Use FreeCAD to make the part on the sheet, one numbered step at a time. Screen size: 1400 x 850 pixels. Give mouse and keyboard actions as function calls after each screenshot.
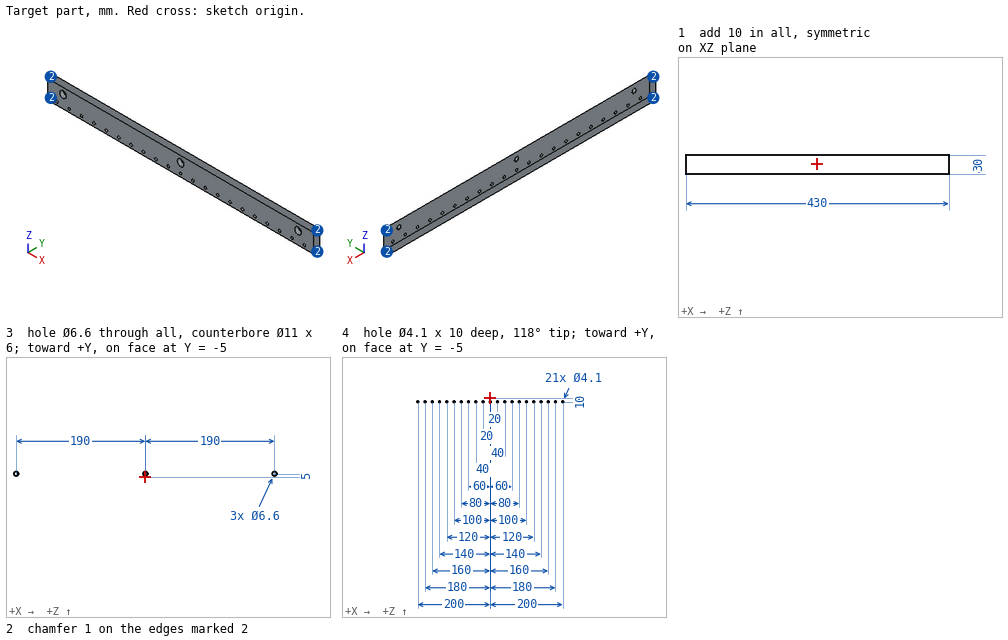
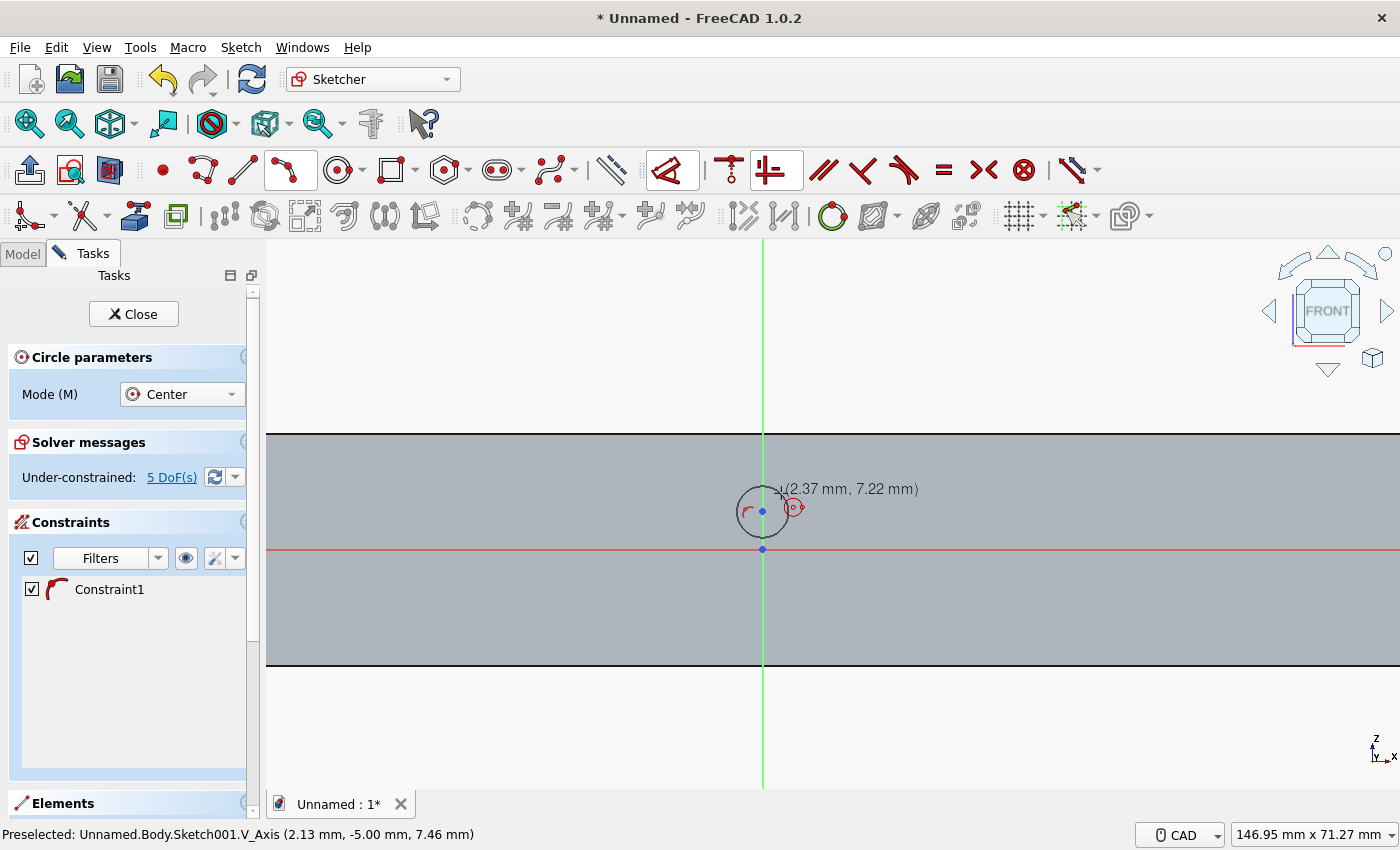
scroll(765, 513, down, 8)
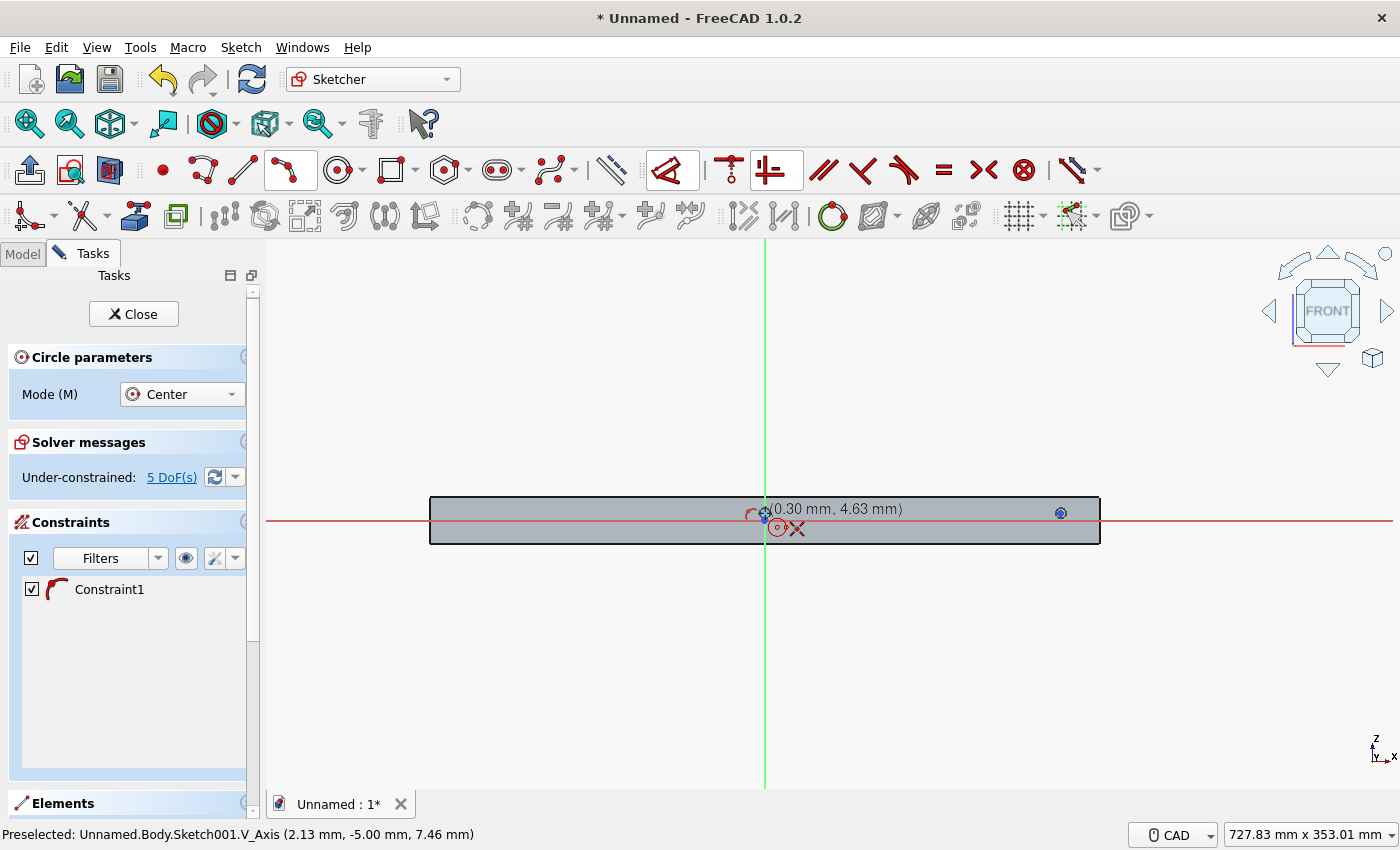
scroll(469, 513, up, 8)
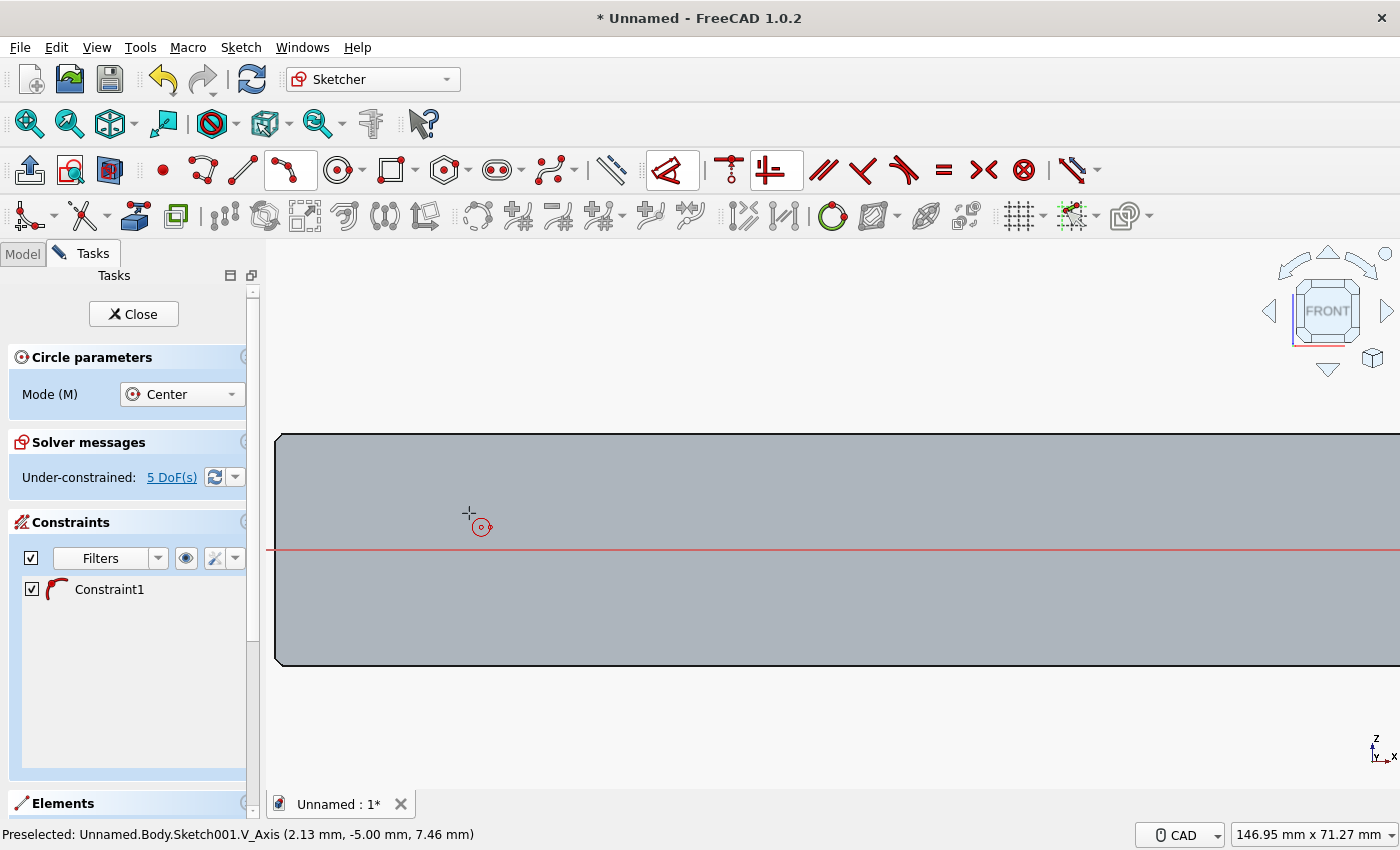
click(468, 511)
click(486, 493)
key(Escape)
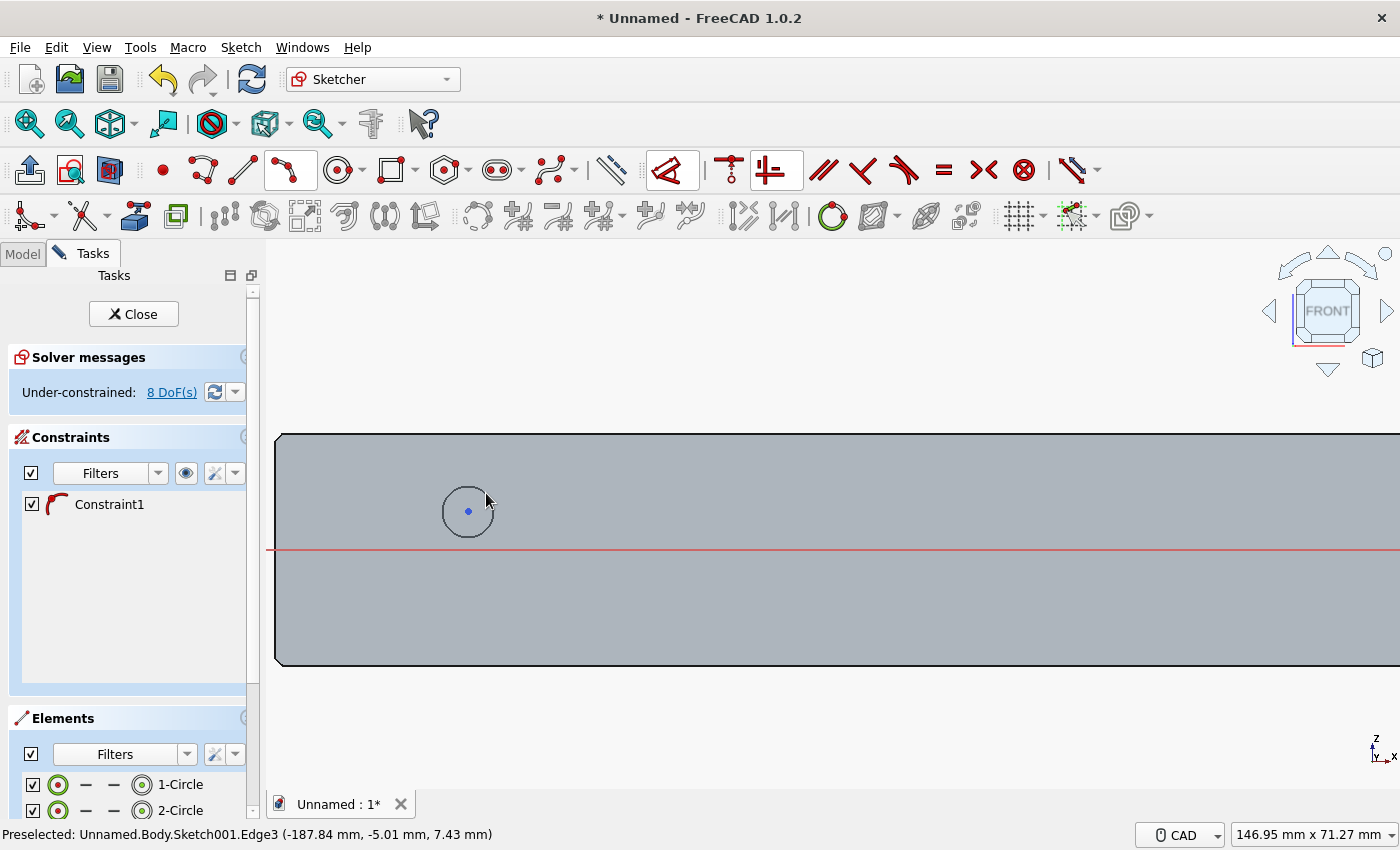
scroll(469, 513, down, 8)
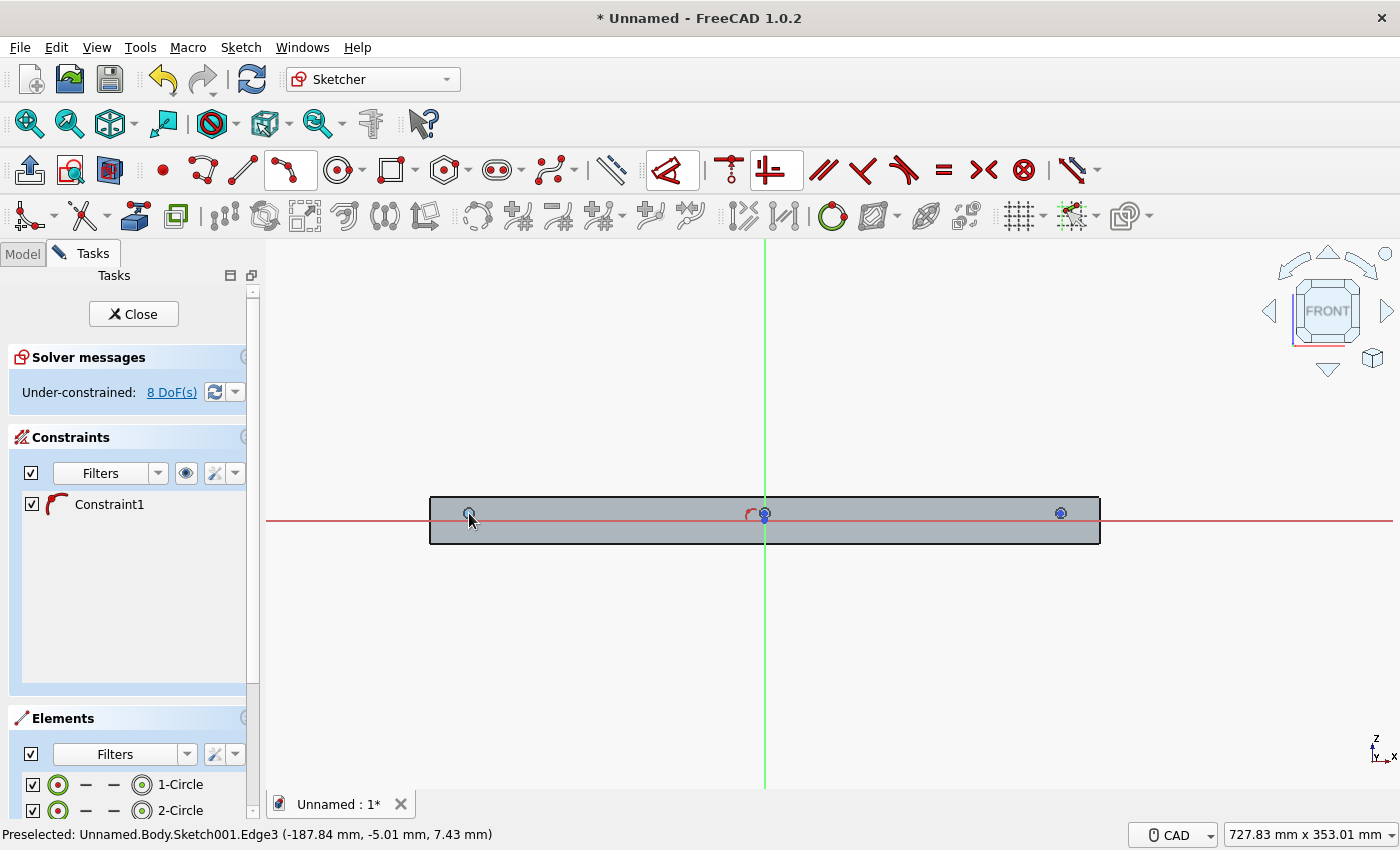
scroll(1065, 510, up, 5)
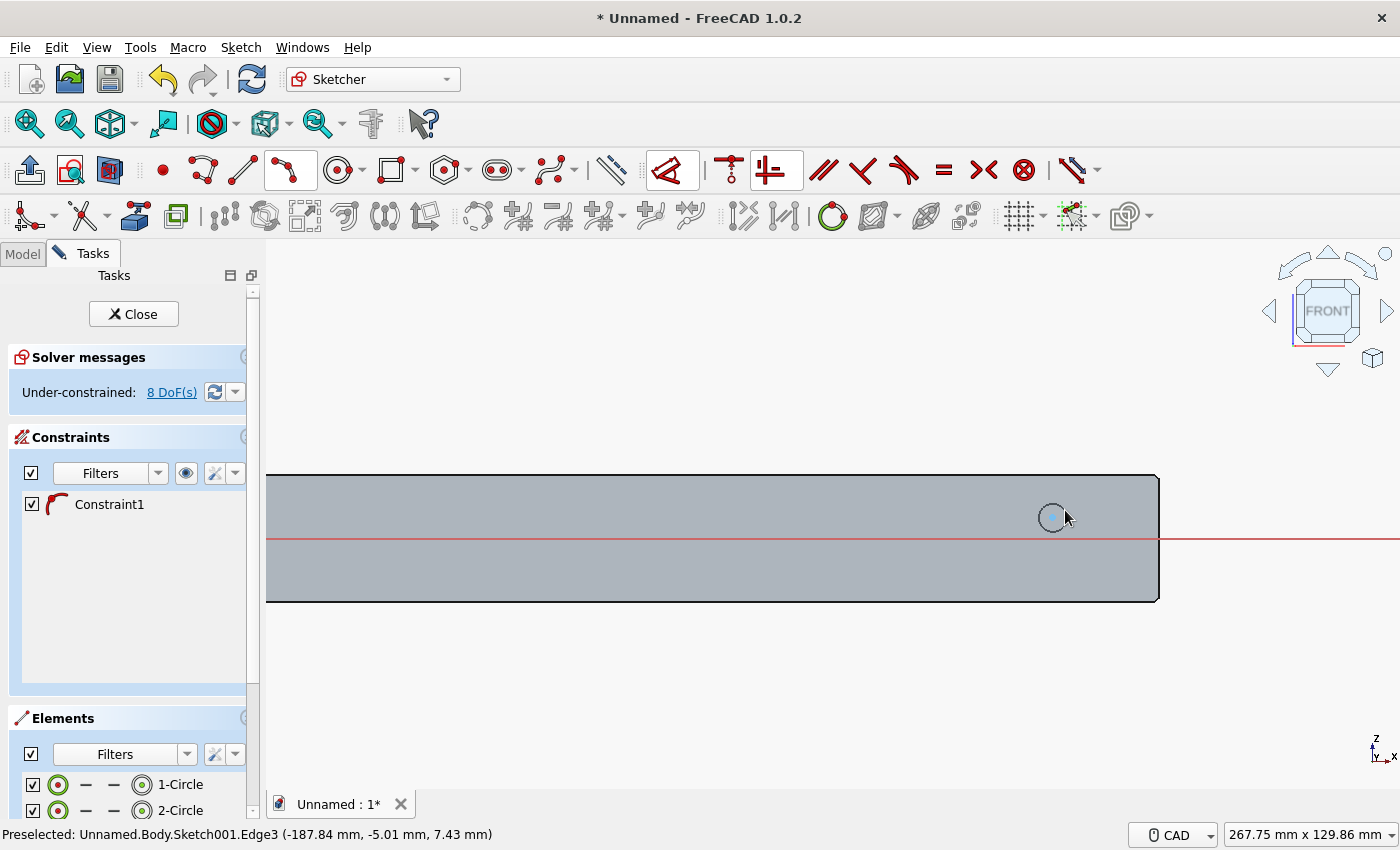
click(1063, 508)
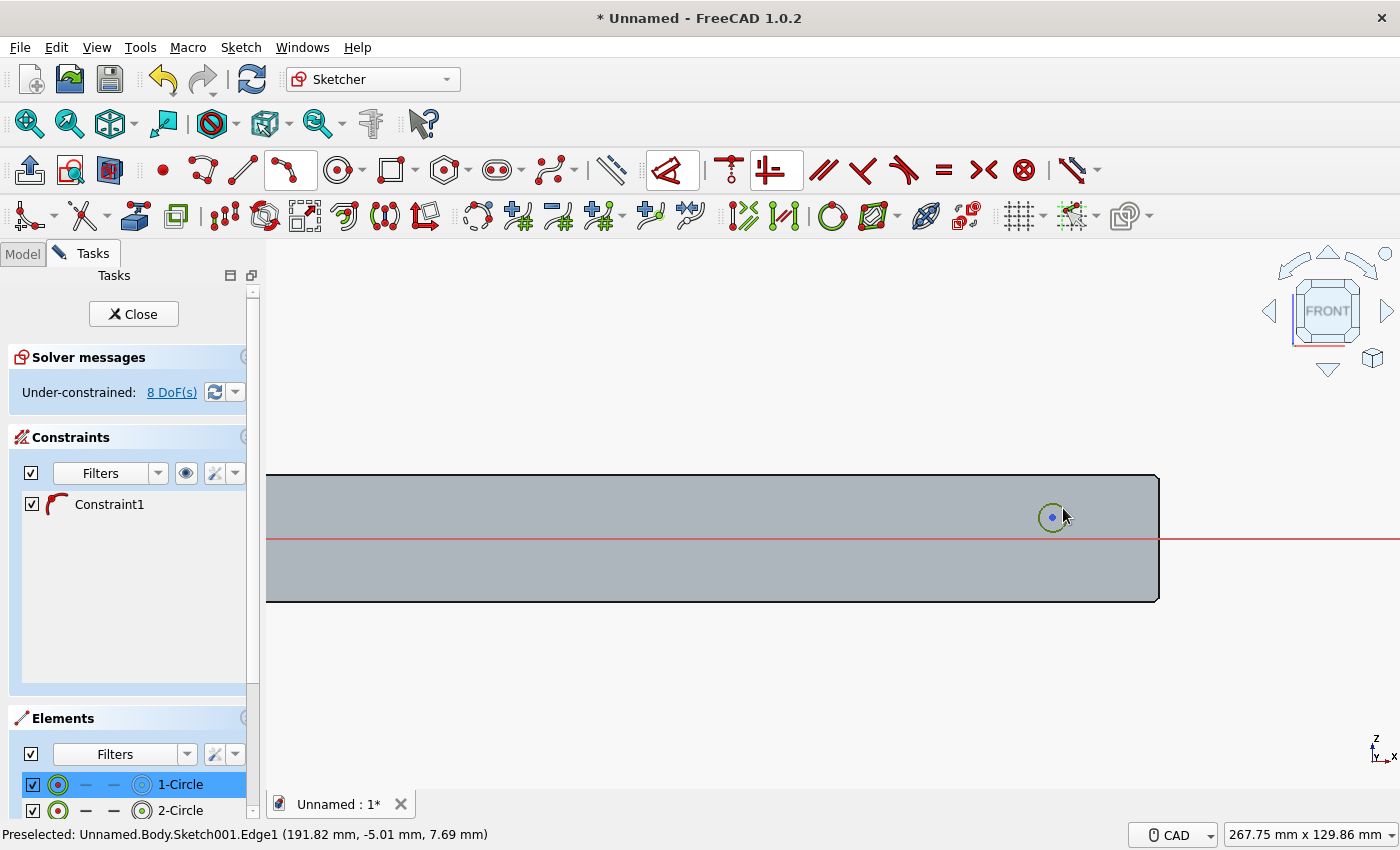
scroll(1065, 510, down, 5)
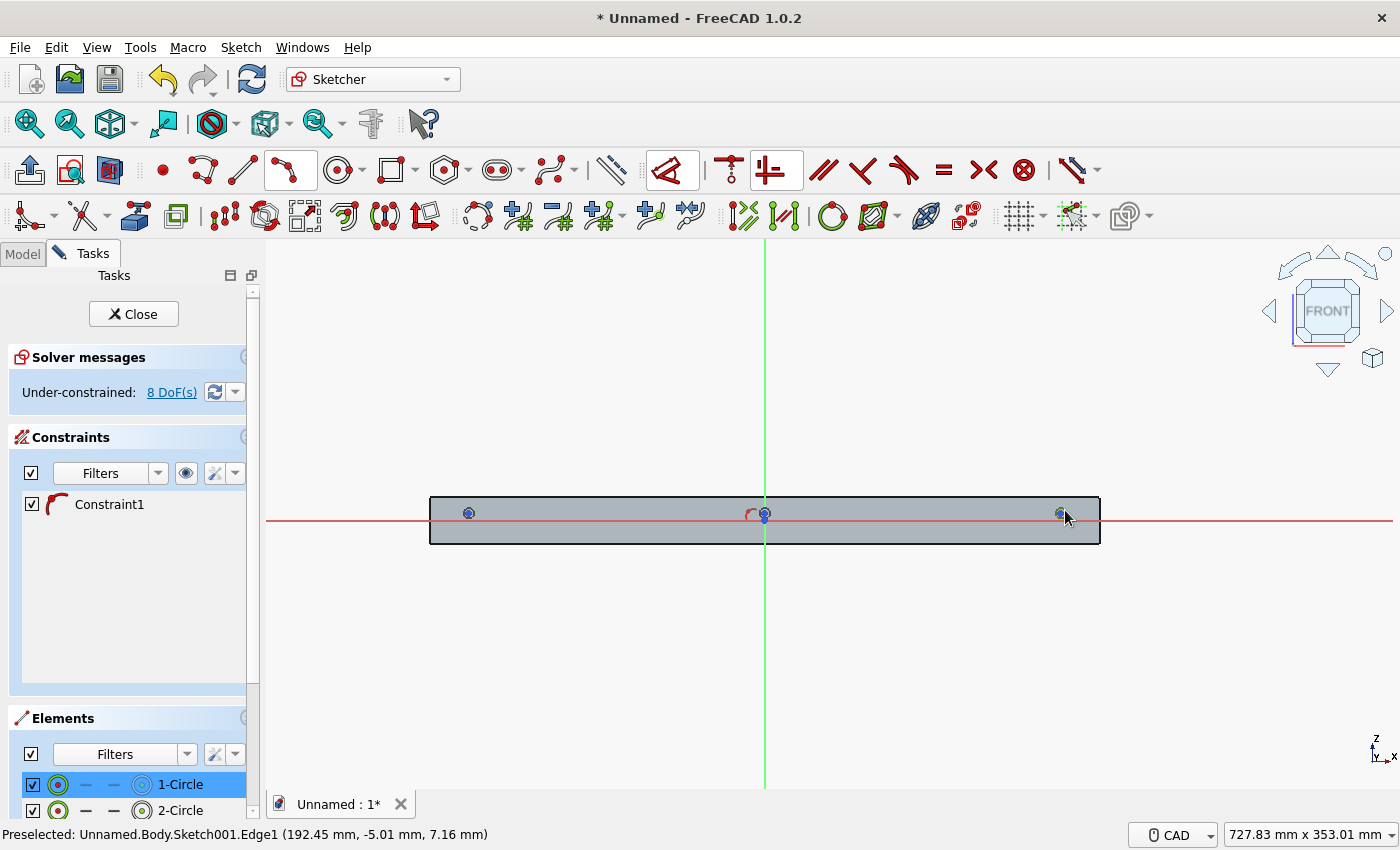
scroll(769, 510, up, 7)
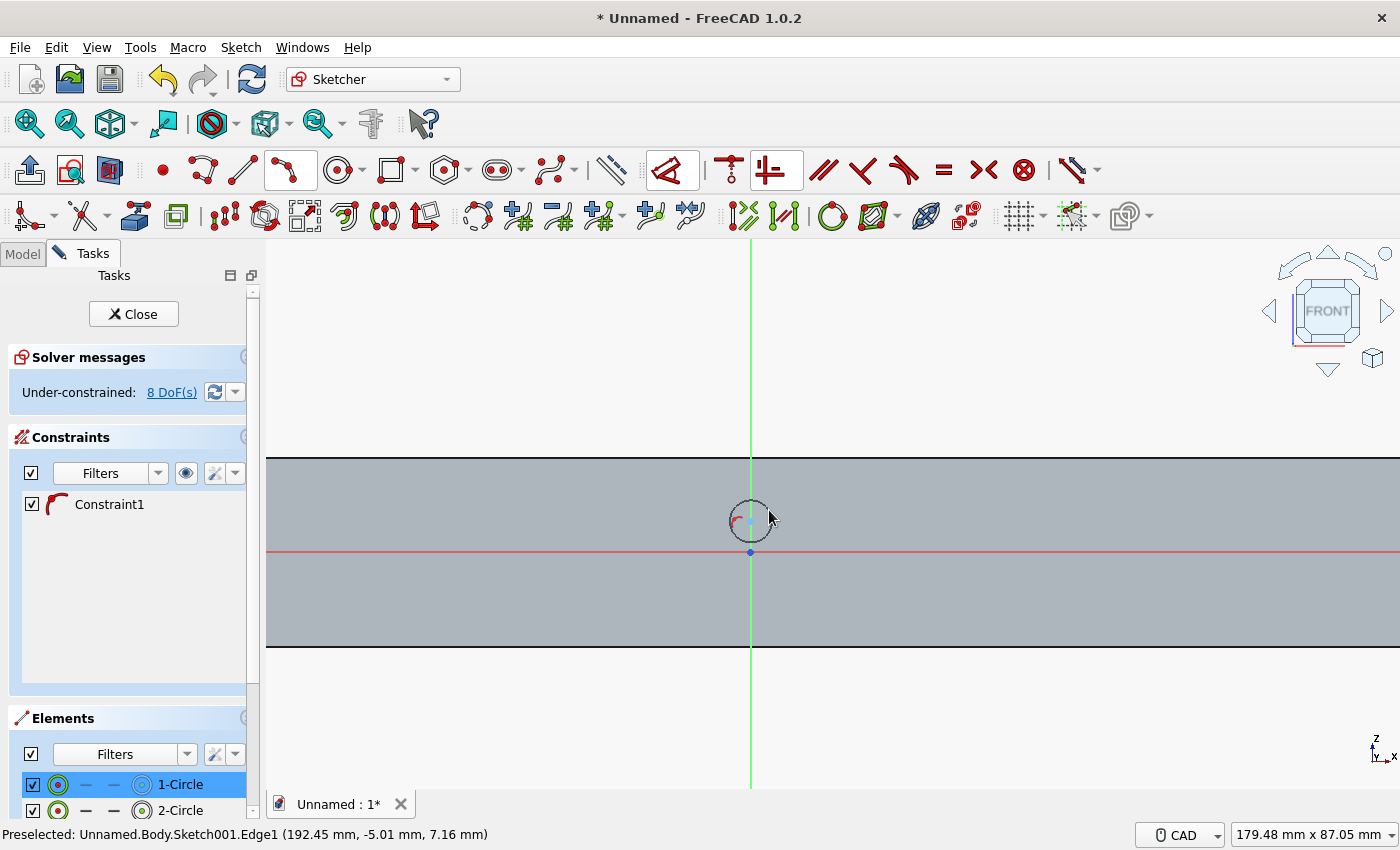
click(766, 507)